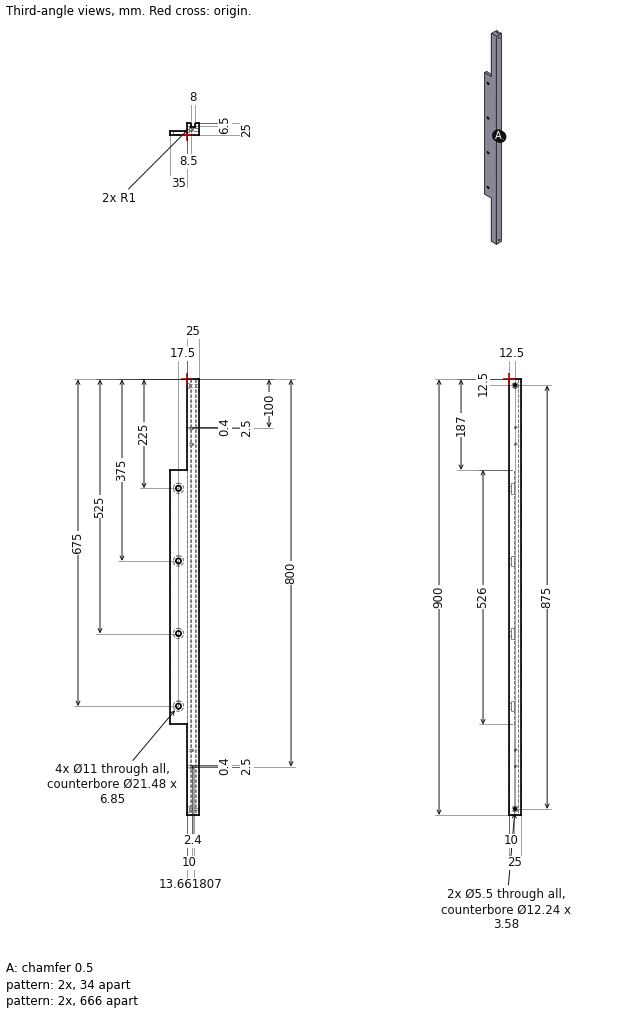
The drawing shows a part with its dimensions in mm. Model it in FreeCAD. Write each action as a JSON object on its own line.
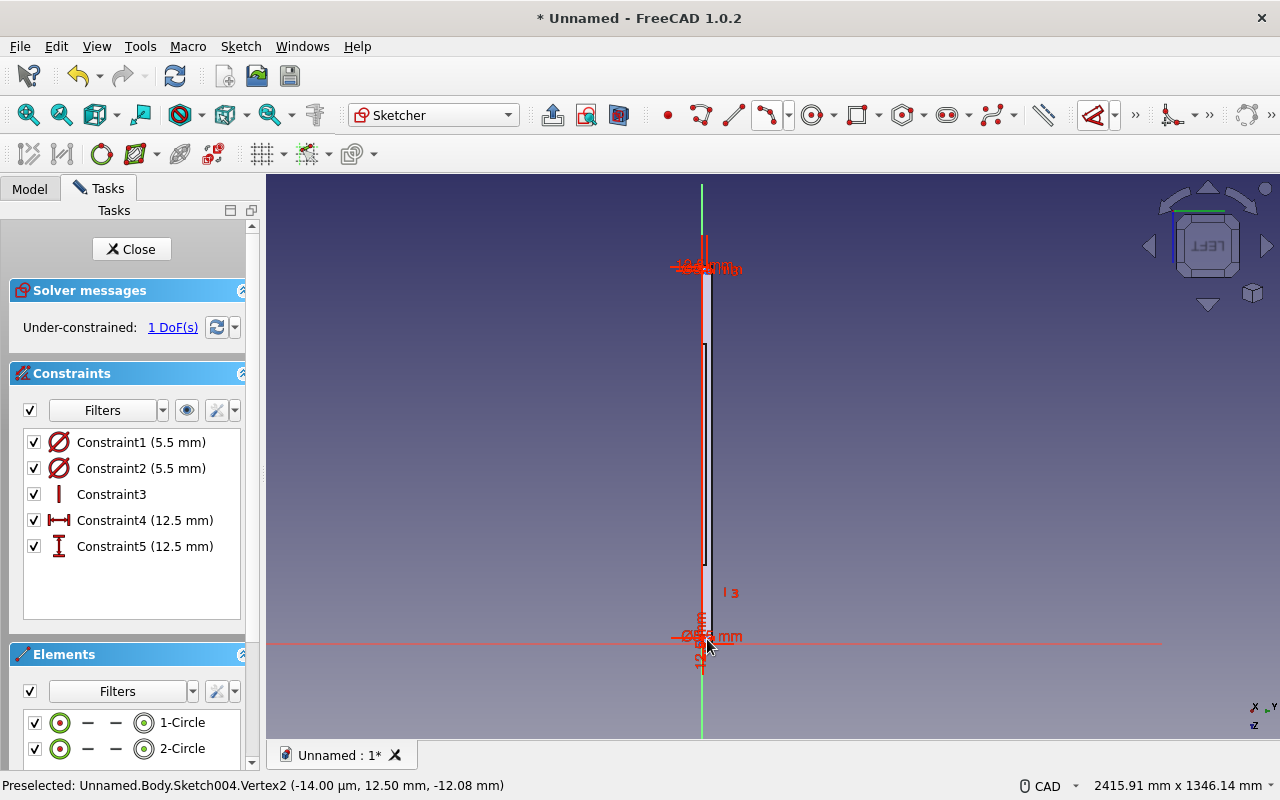
{"action": "left_click", "coordinate": [707, 271]}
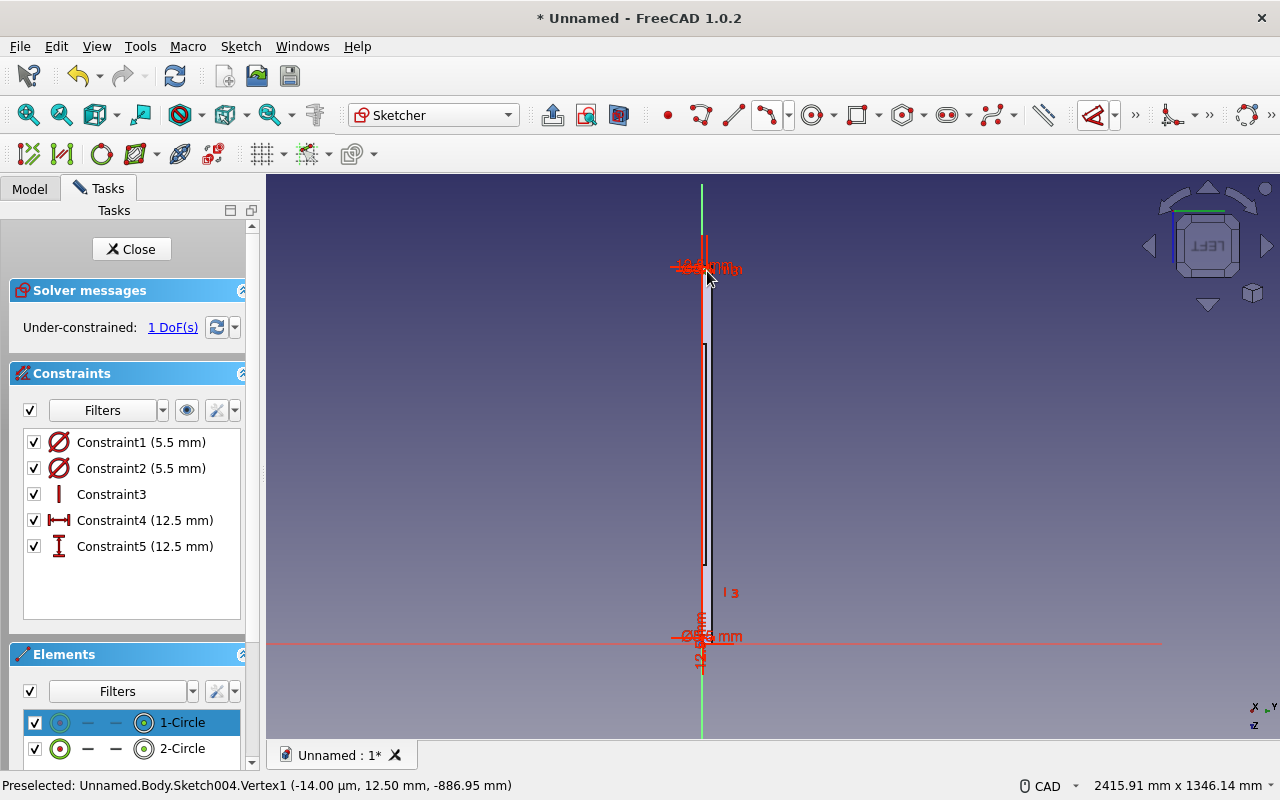
{"action": "scroll", "coordinate": [707, 638], "scroll_direction": "up", "scroll_amount": 3}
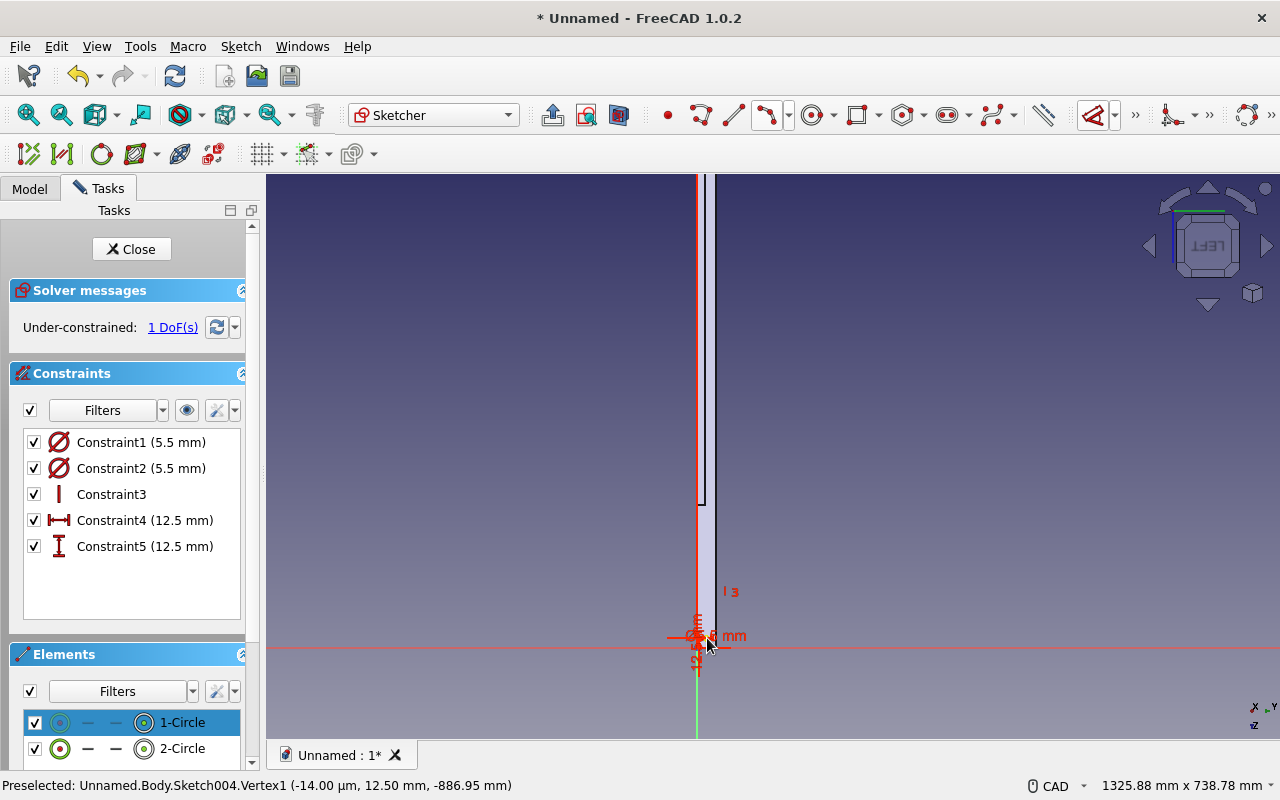
{"action": "left_click", "coordinate": [707, 638]}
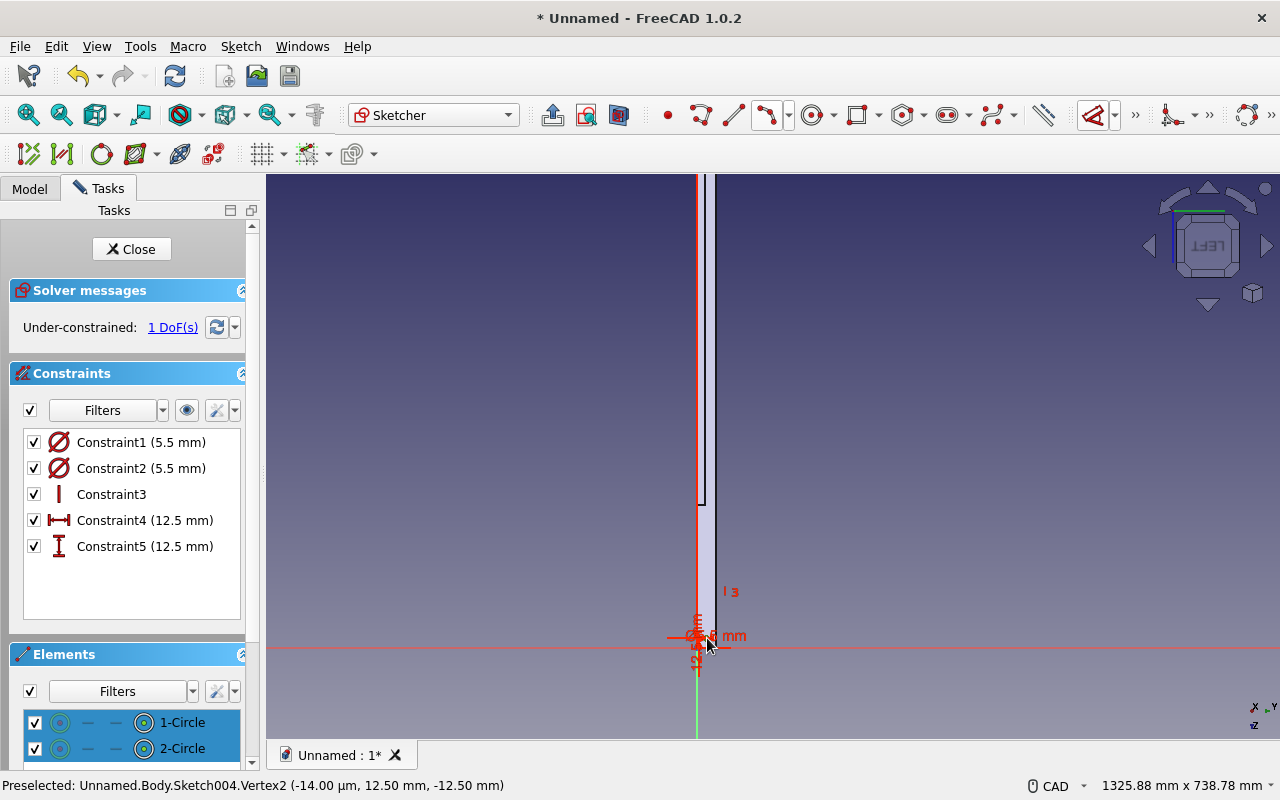
{"action": "key", "text": "i"}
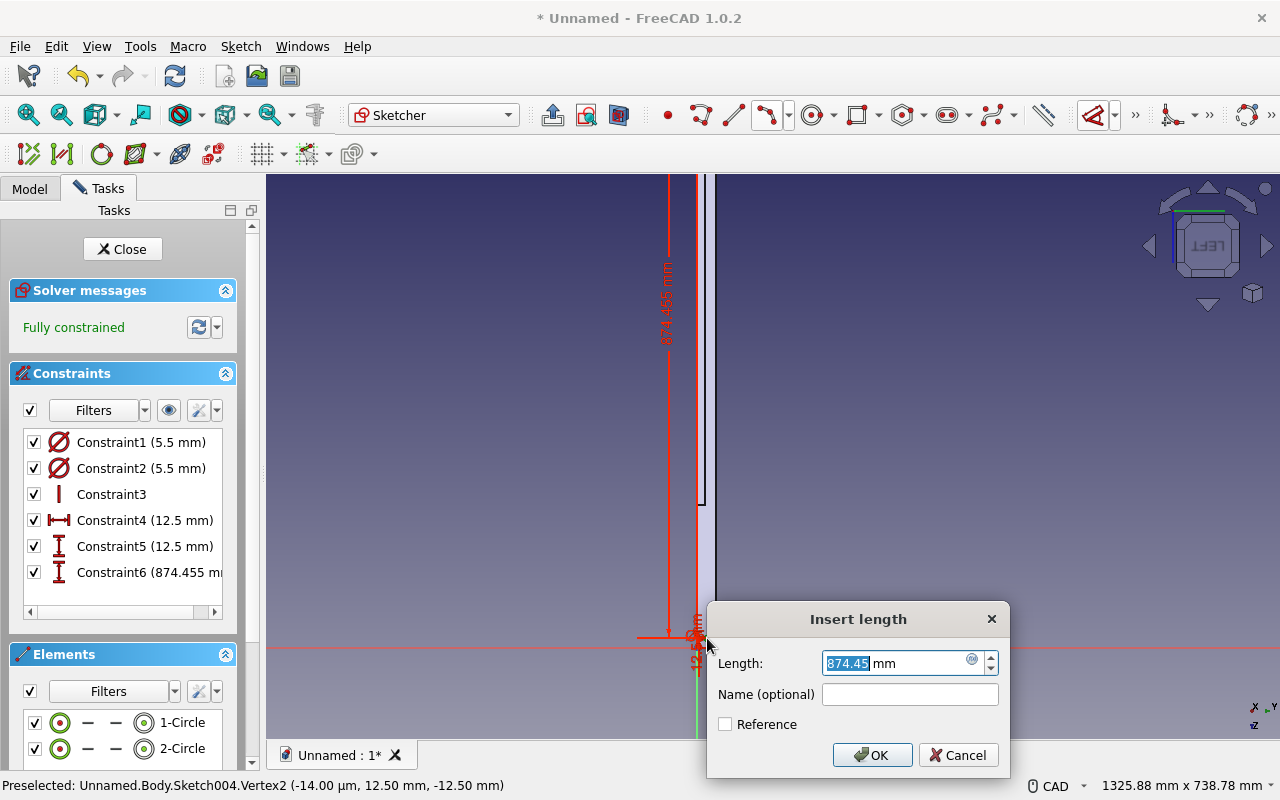
{"action": "type", "text": "875"}
{"action": "key", "text": "Return"}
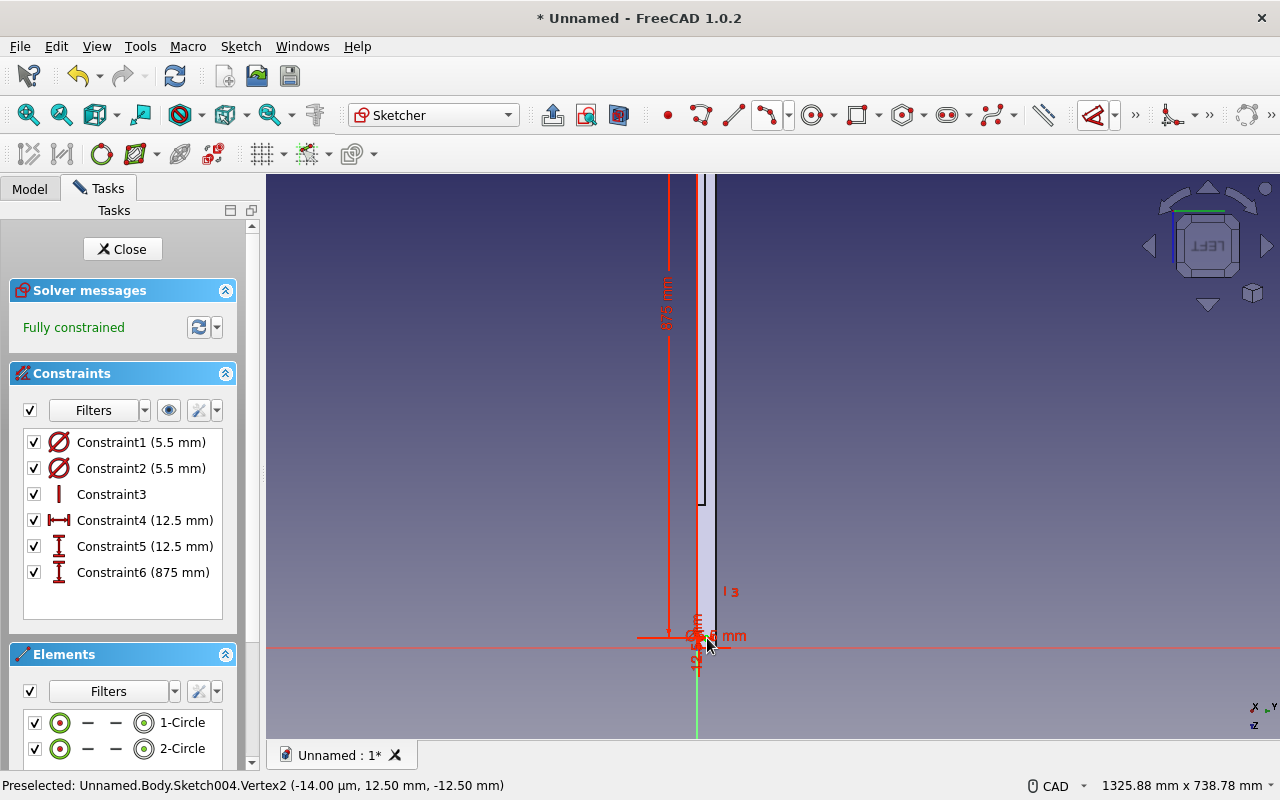
{"action": "left_click", "coordinate": [123, 249]}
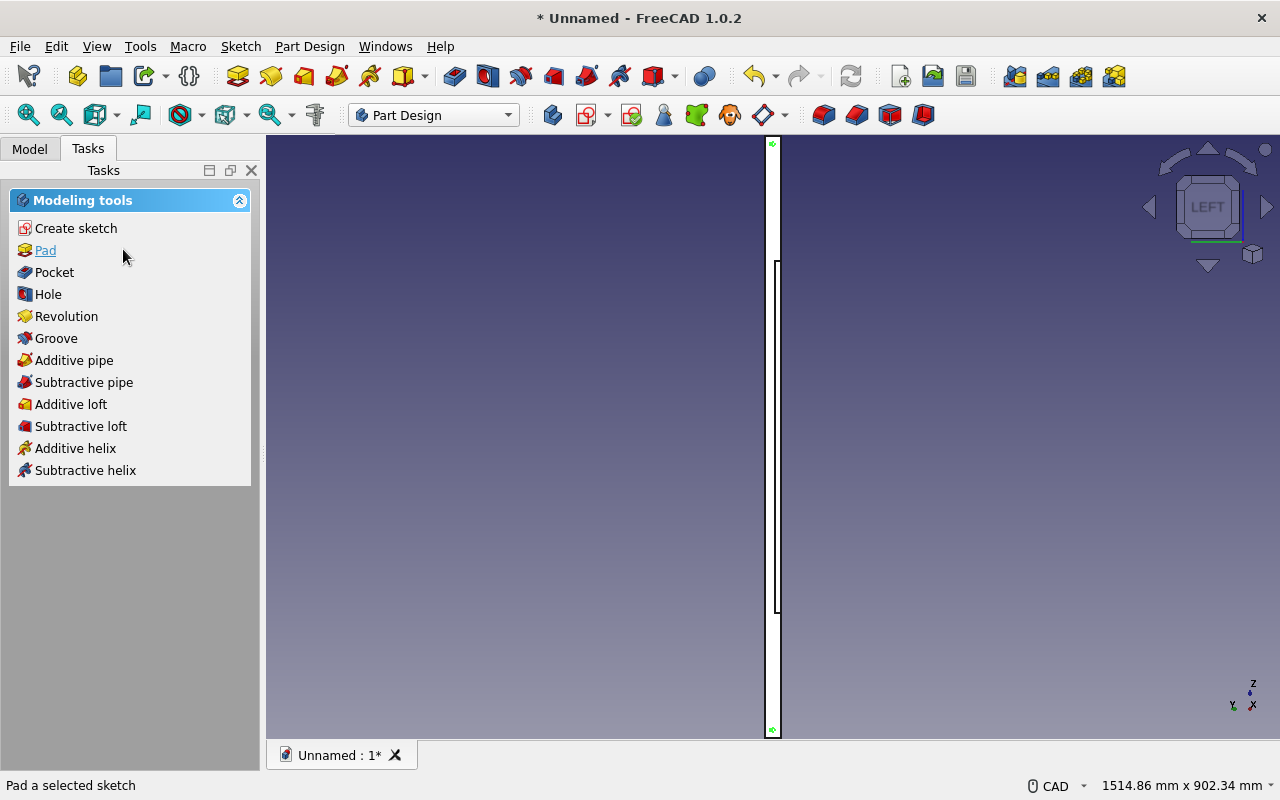
{"action": "left_click", "coordinate": [488, 76]}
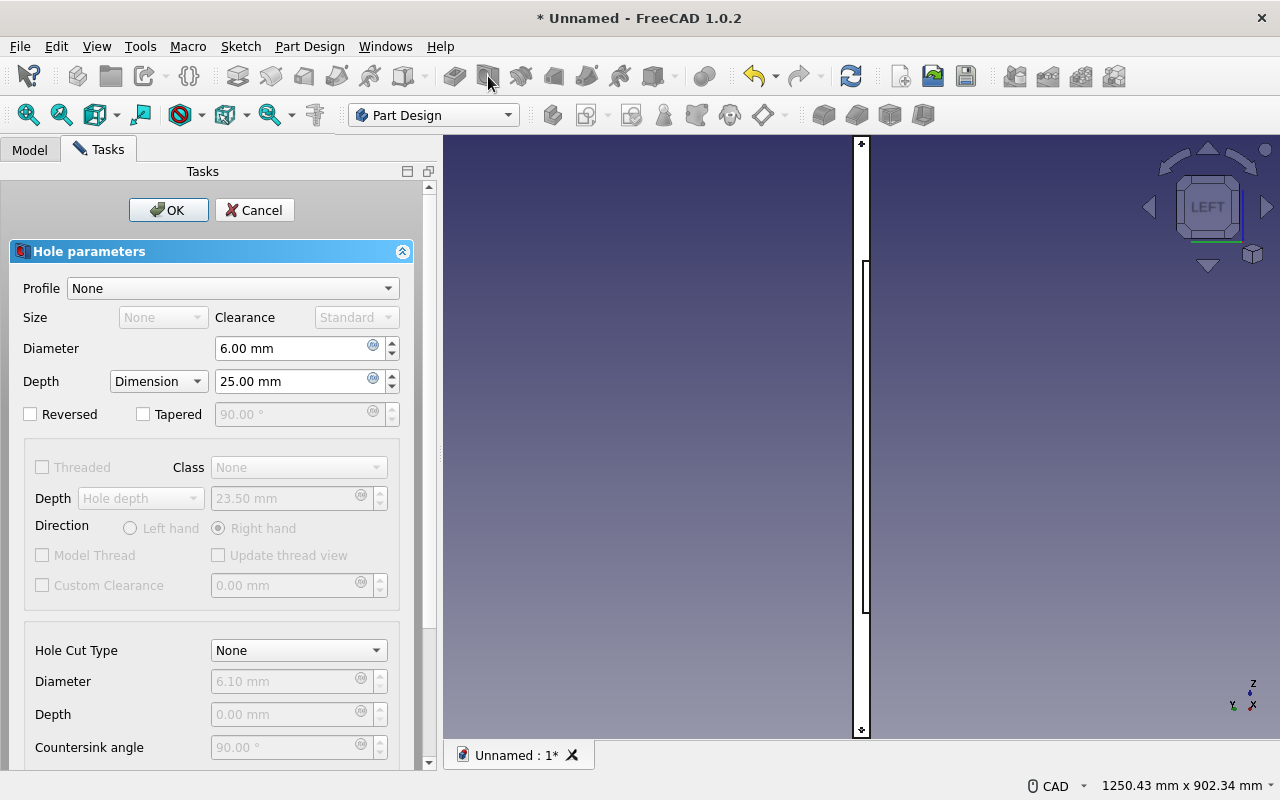
{"action": "triple_click", "coordinate": [300, 348]}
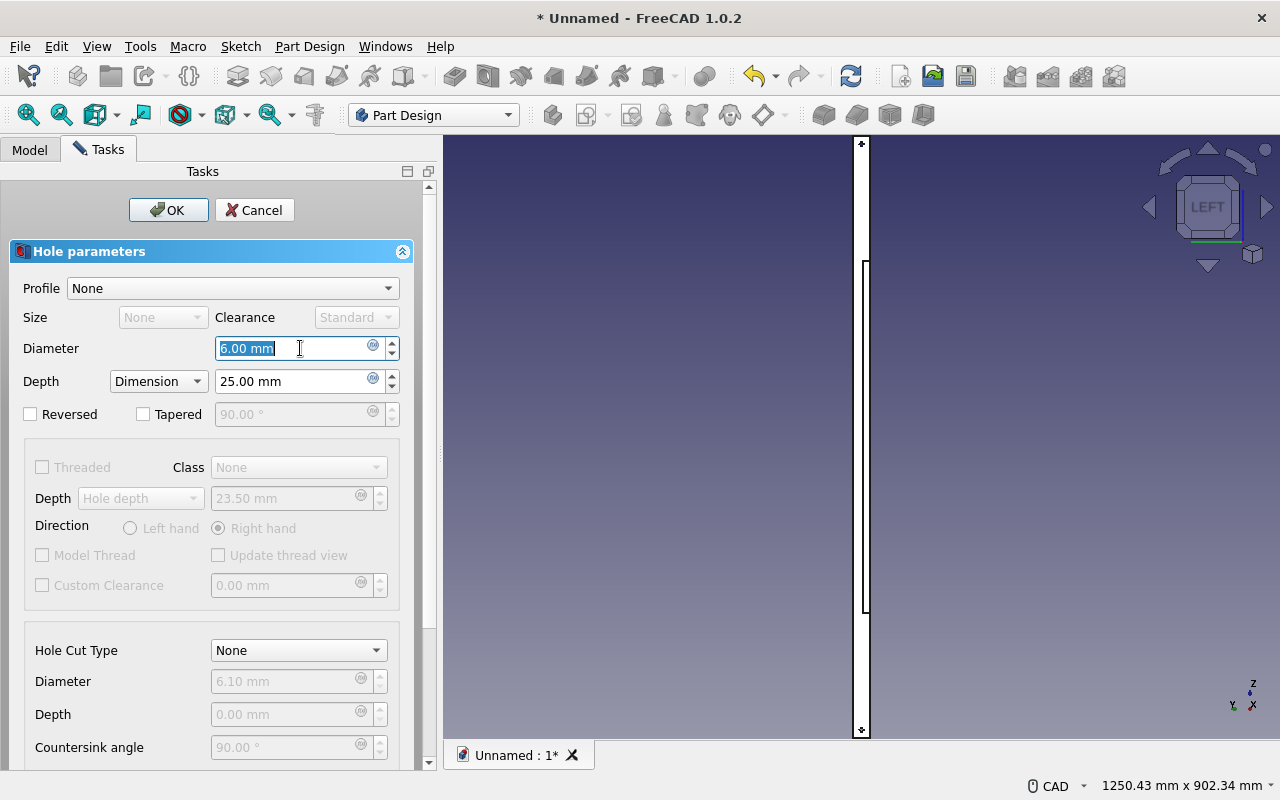
{"action": "type", "text": "5.5"}
{"action": "key", "text": "Tab"}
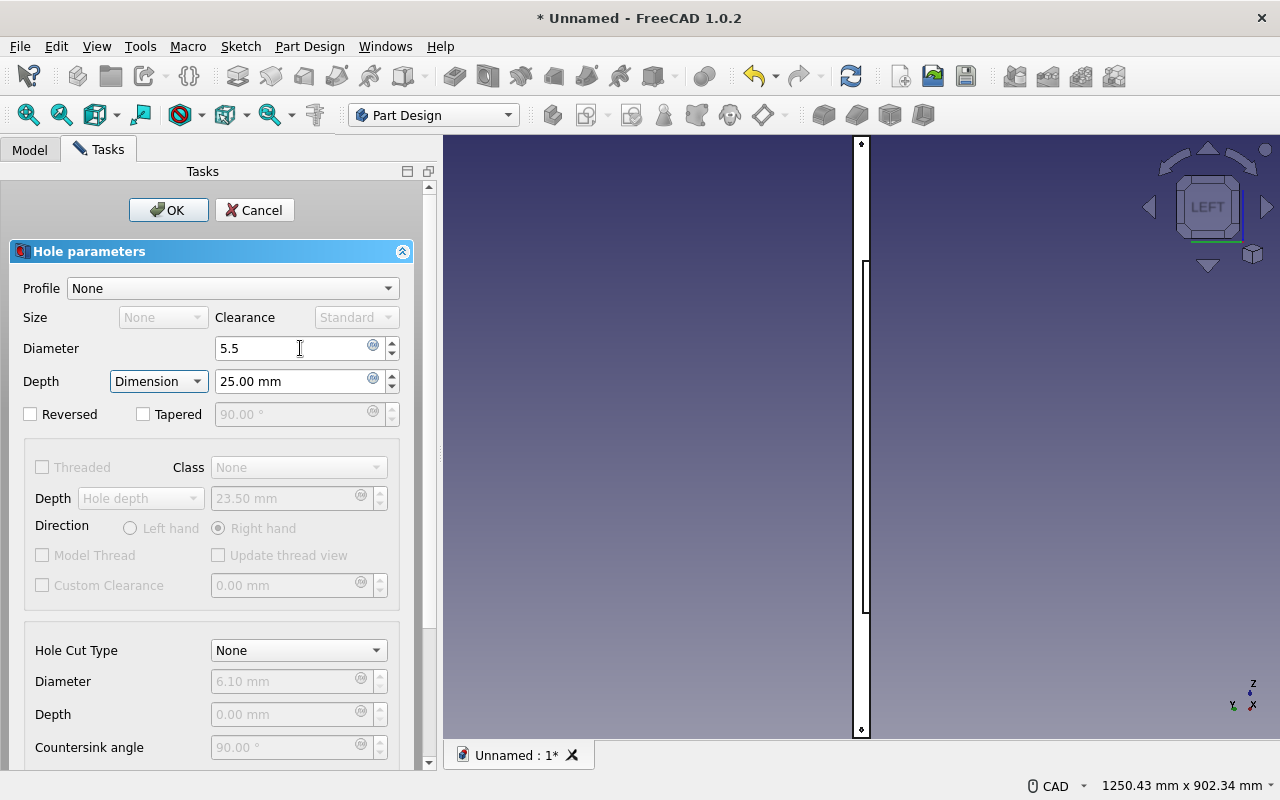
{"action": "left_click", "coordinate": [160, 382]}